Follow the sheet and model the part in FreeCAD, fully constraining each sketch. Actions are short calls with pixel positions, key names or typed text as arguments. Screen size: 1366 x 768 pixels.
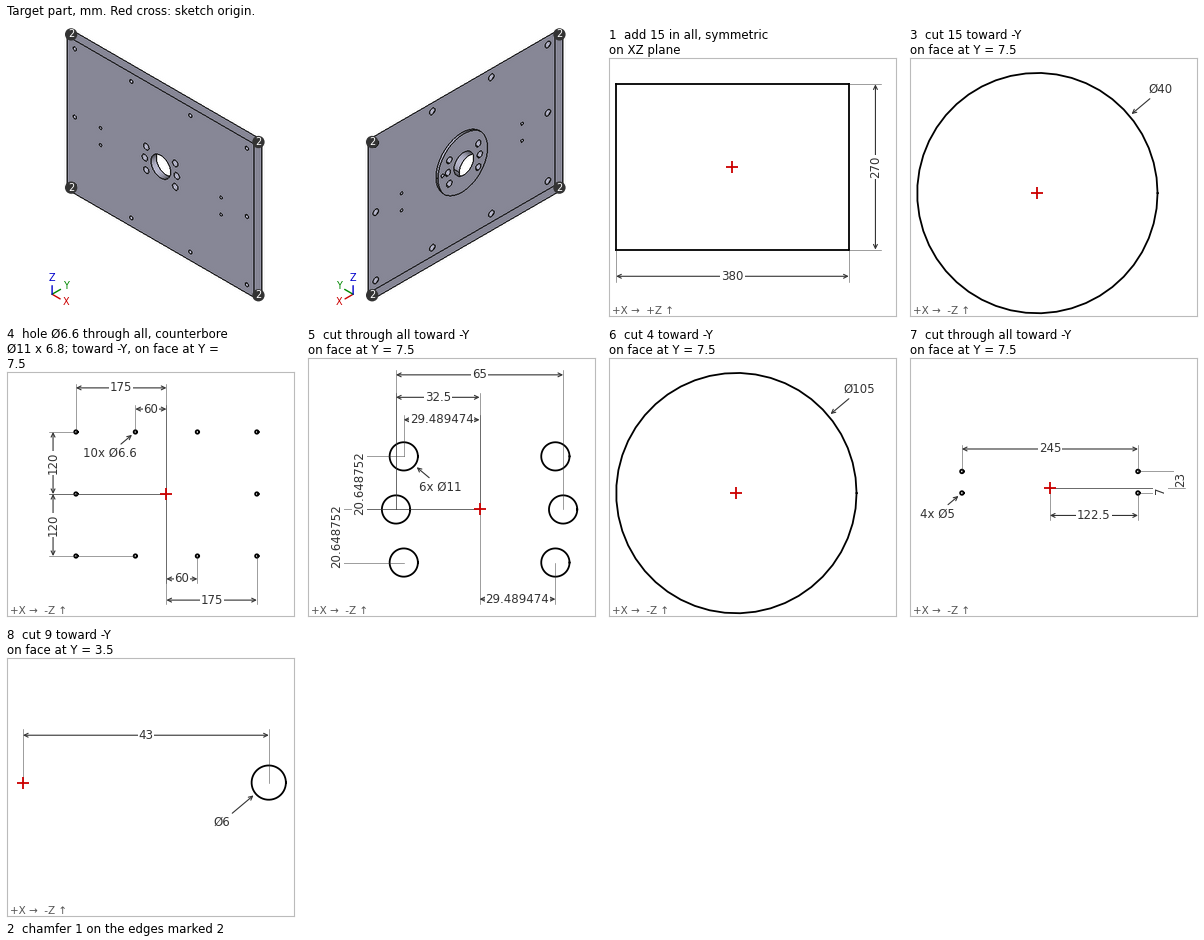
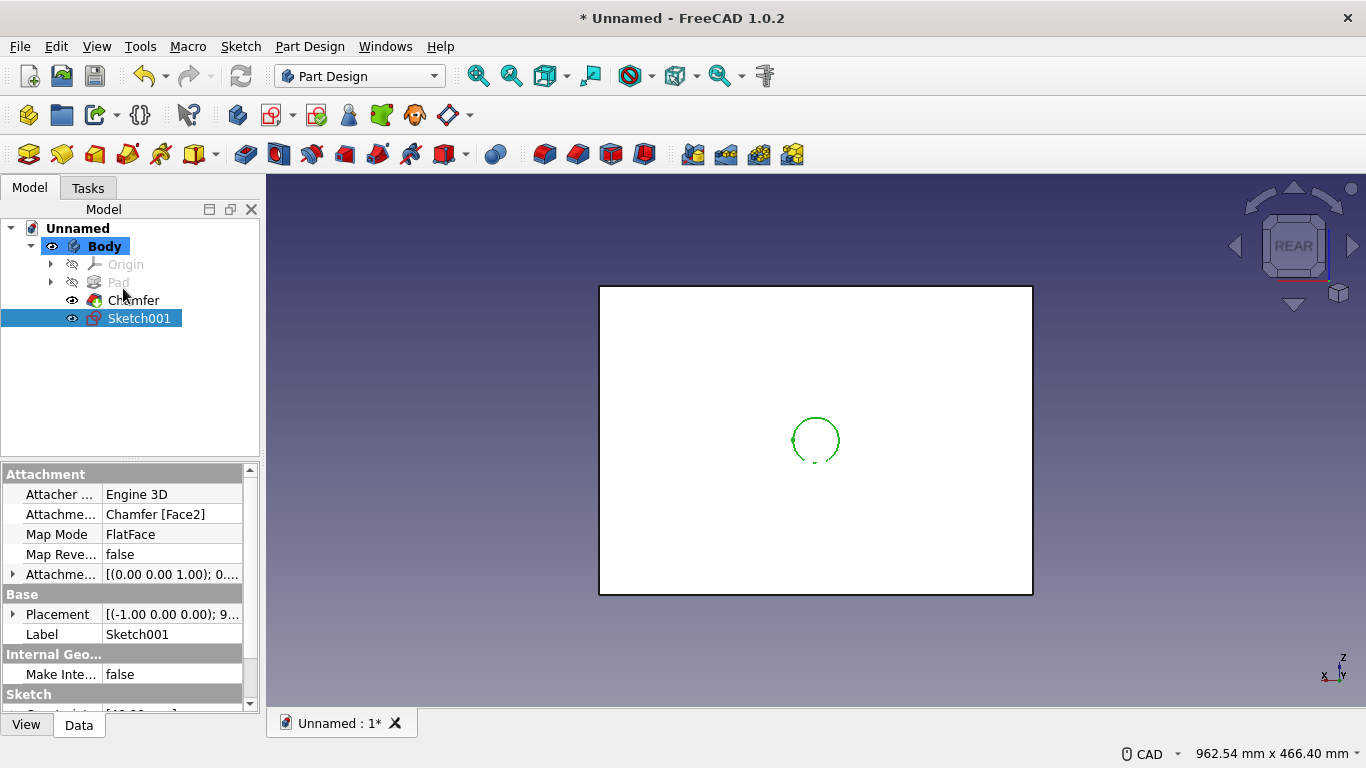
click(246, 154)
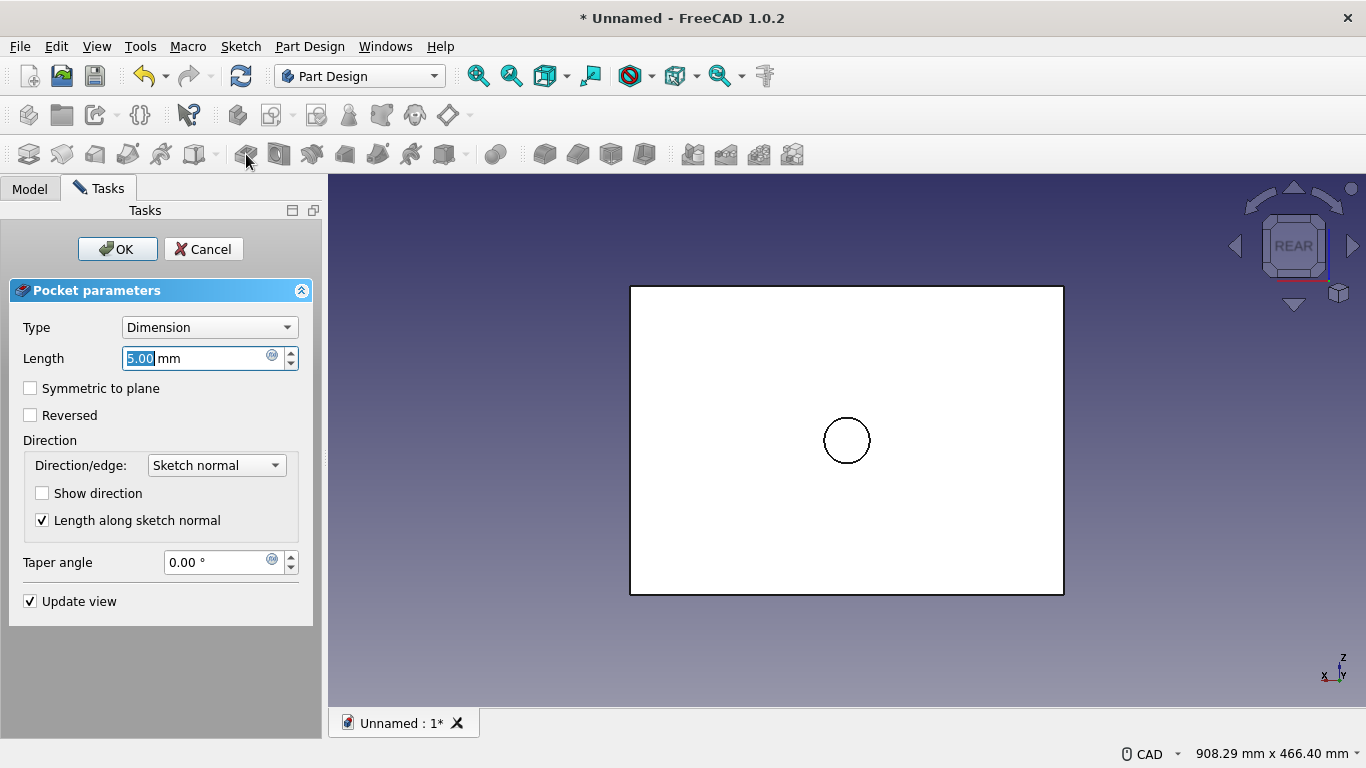
text(15)
key(Tab)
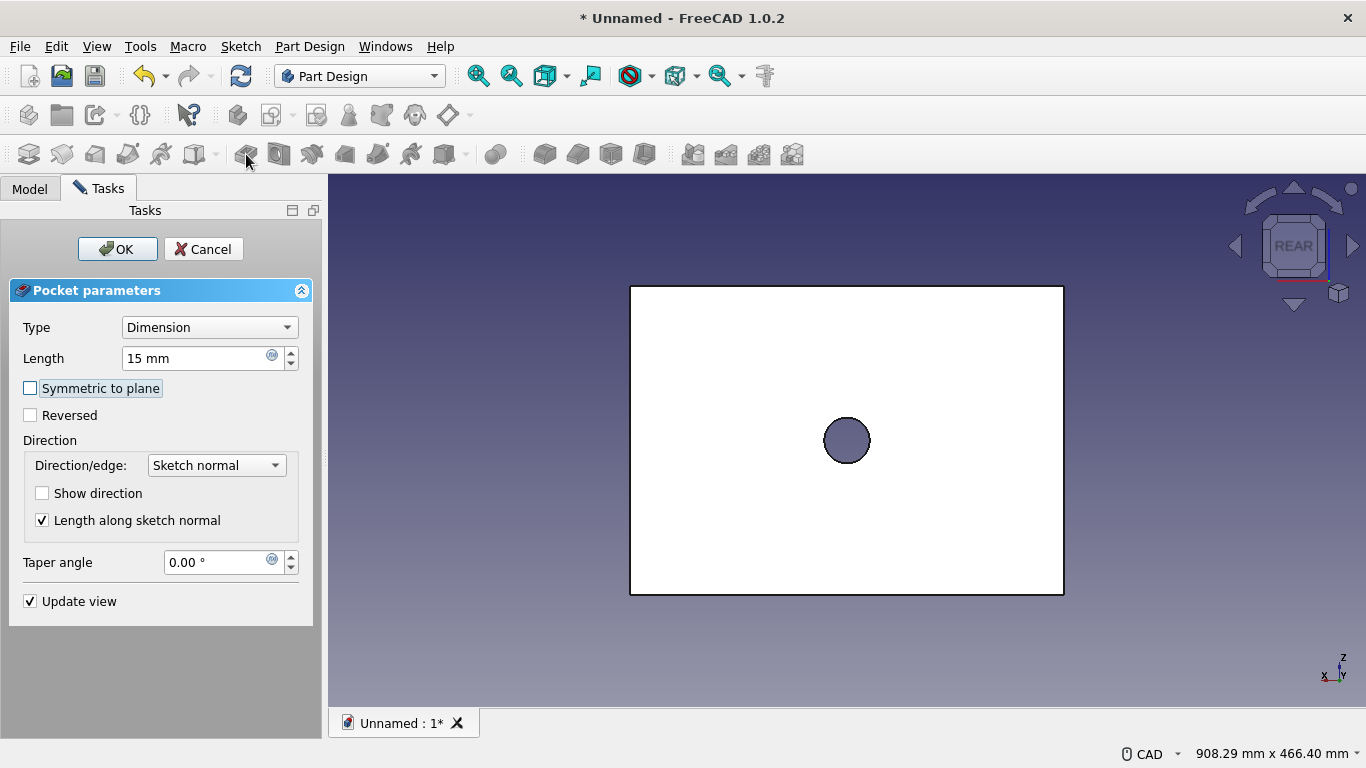
click(118, 249)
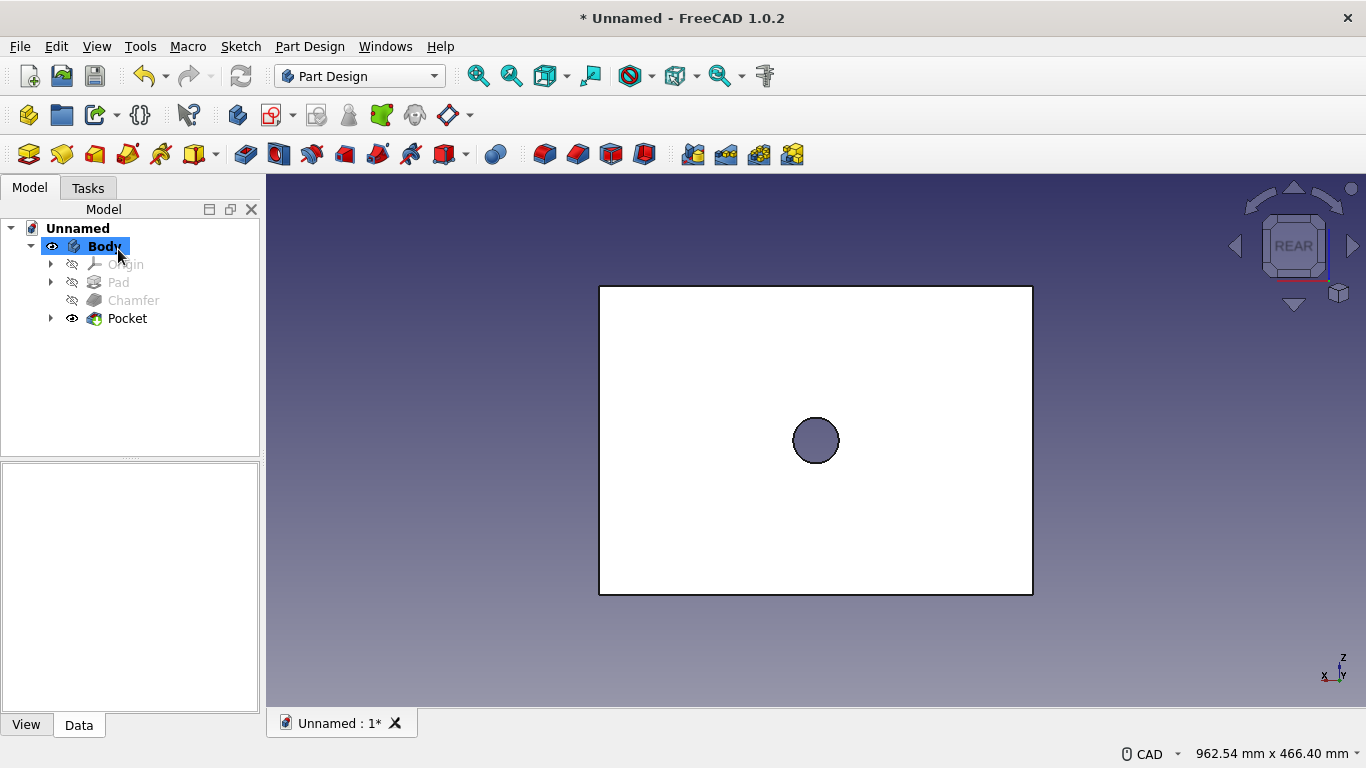
click(692, 395)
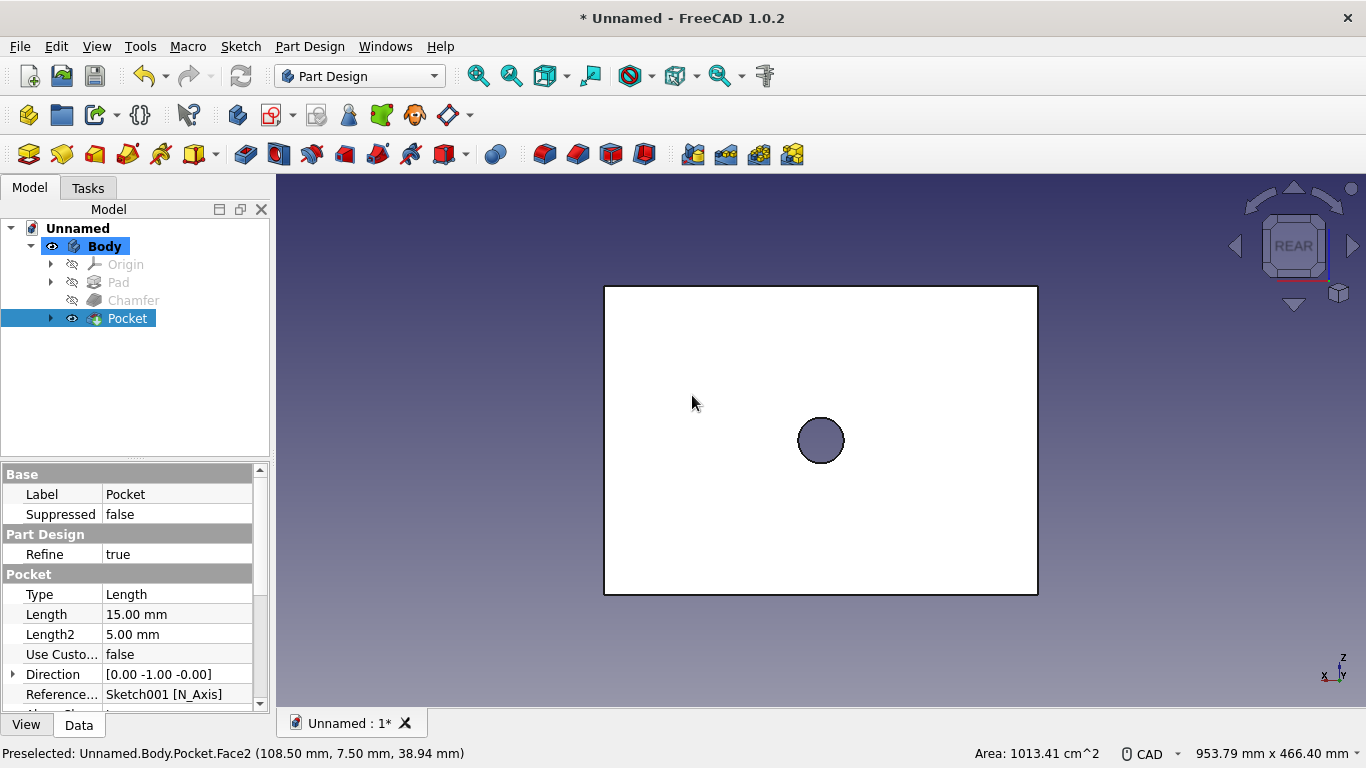
click(270, 116)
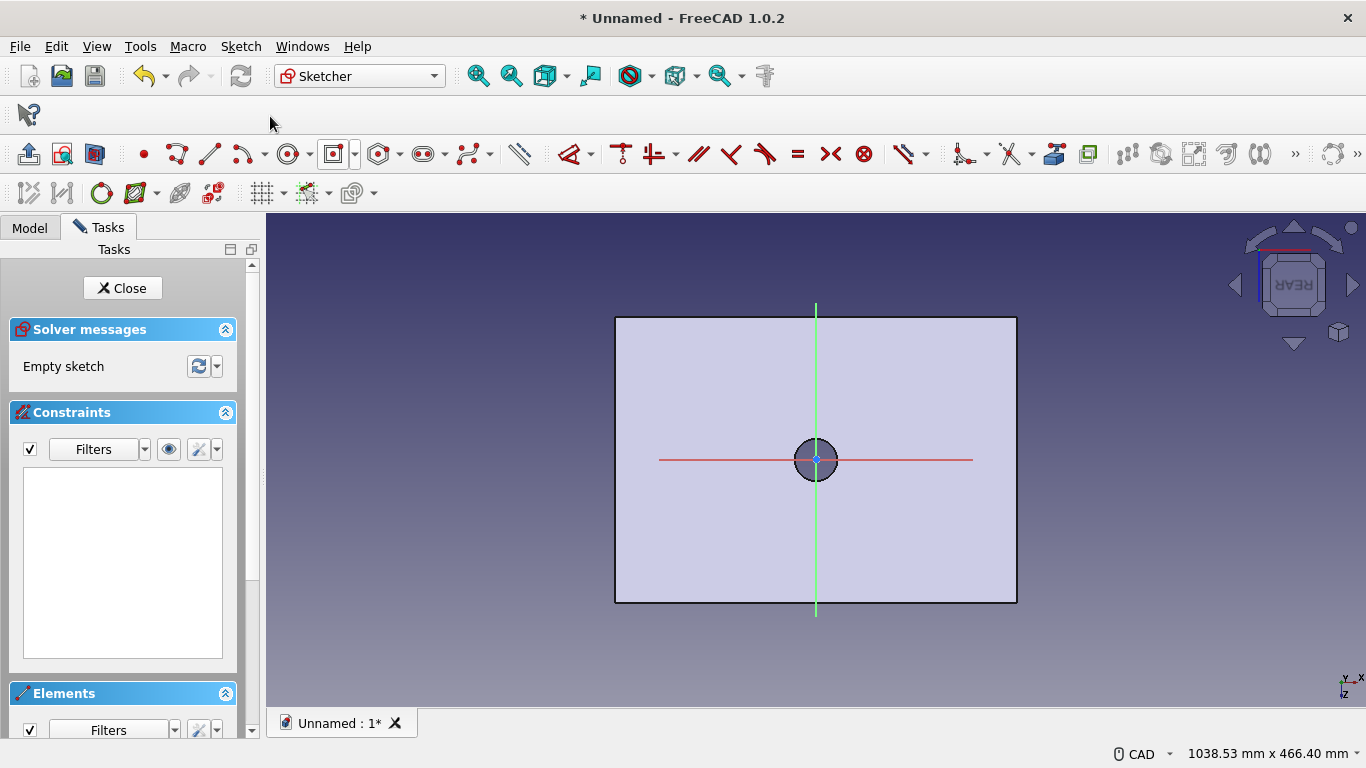
click(288, 154)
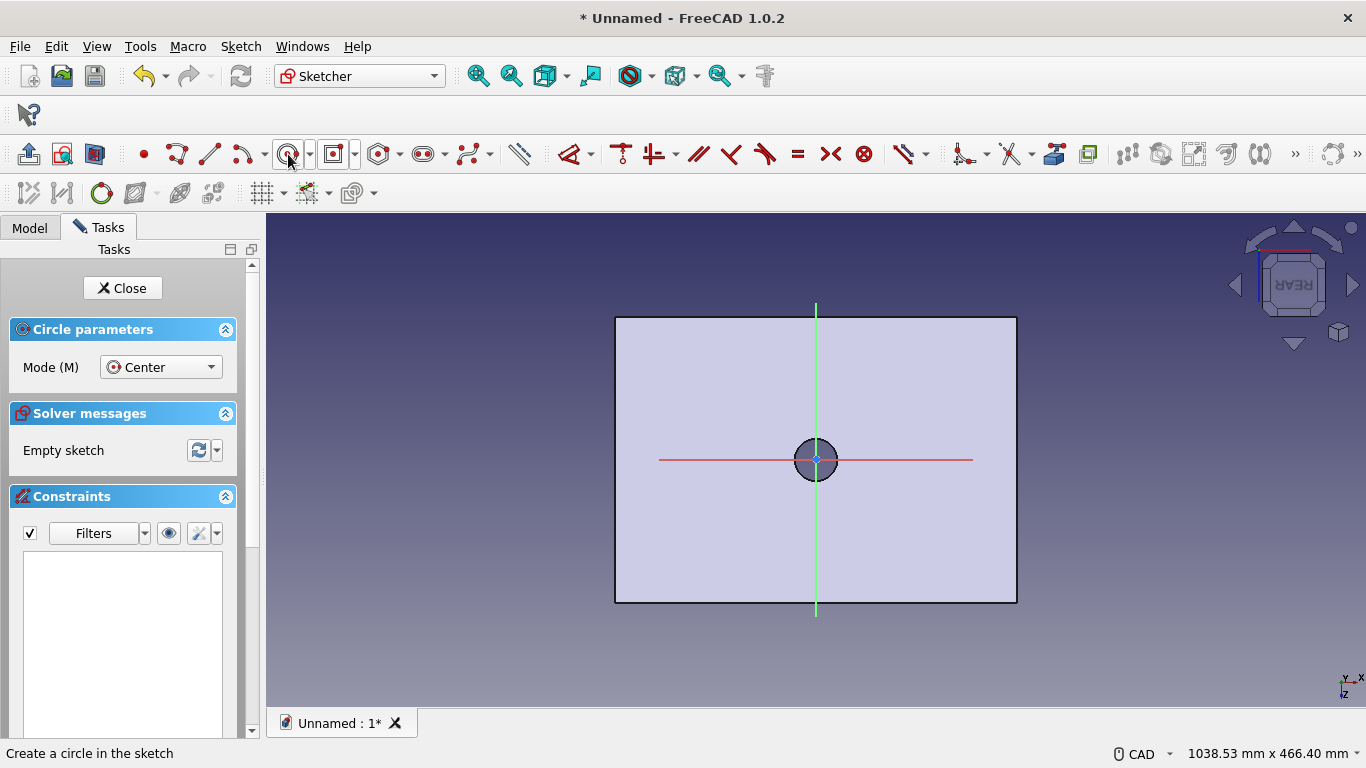
scroll(631, 333, up, 10)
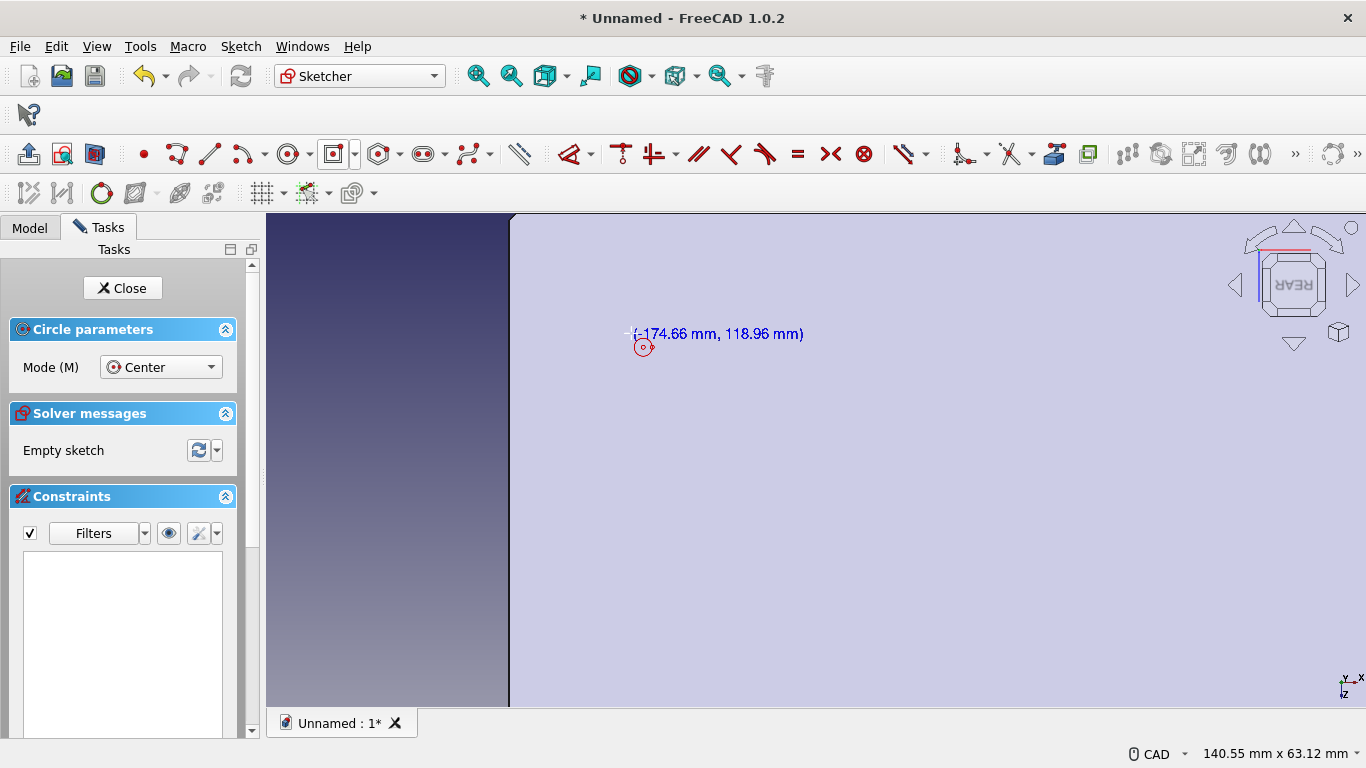
scroll(500, 300, down, 9)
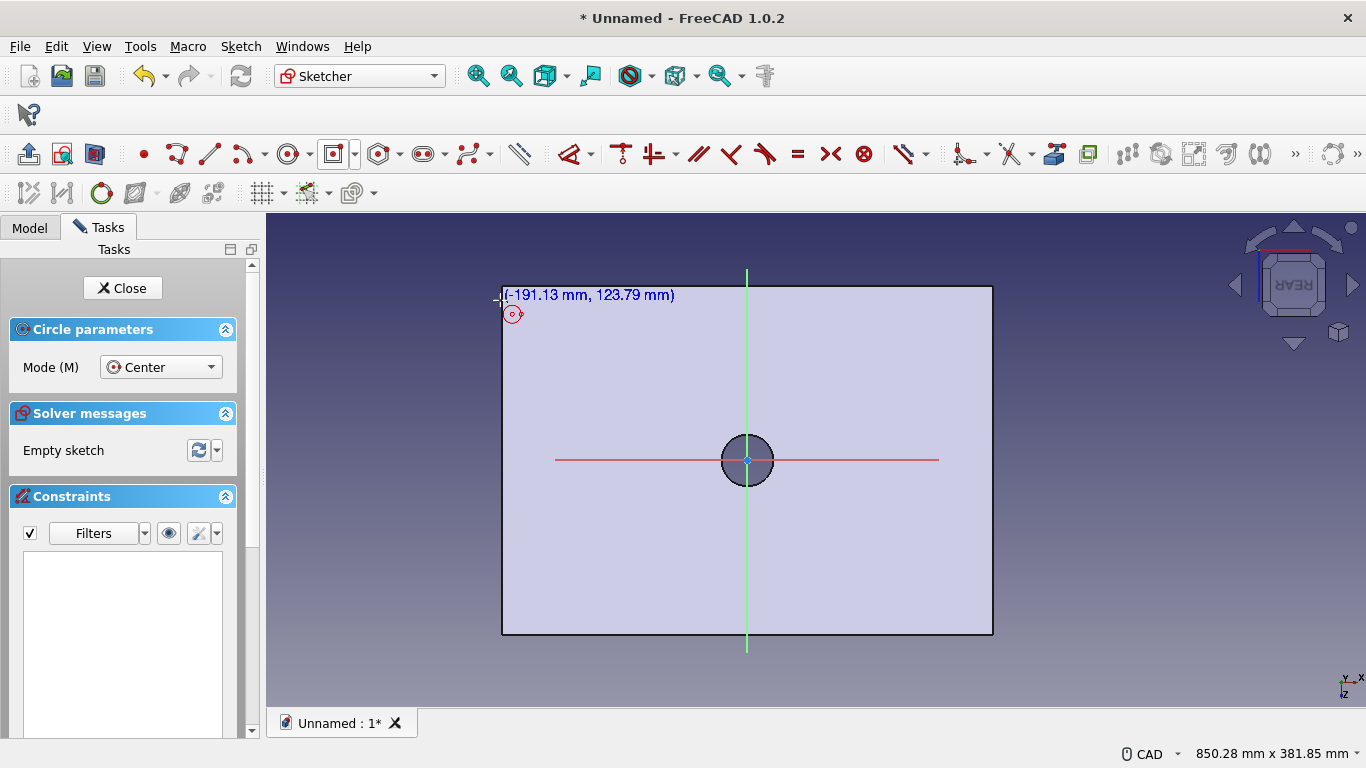
click(521, 305)